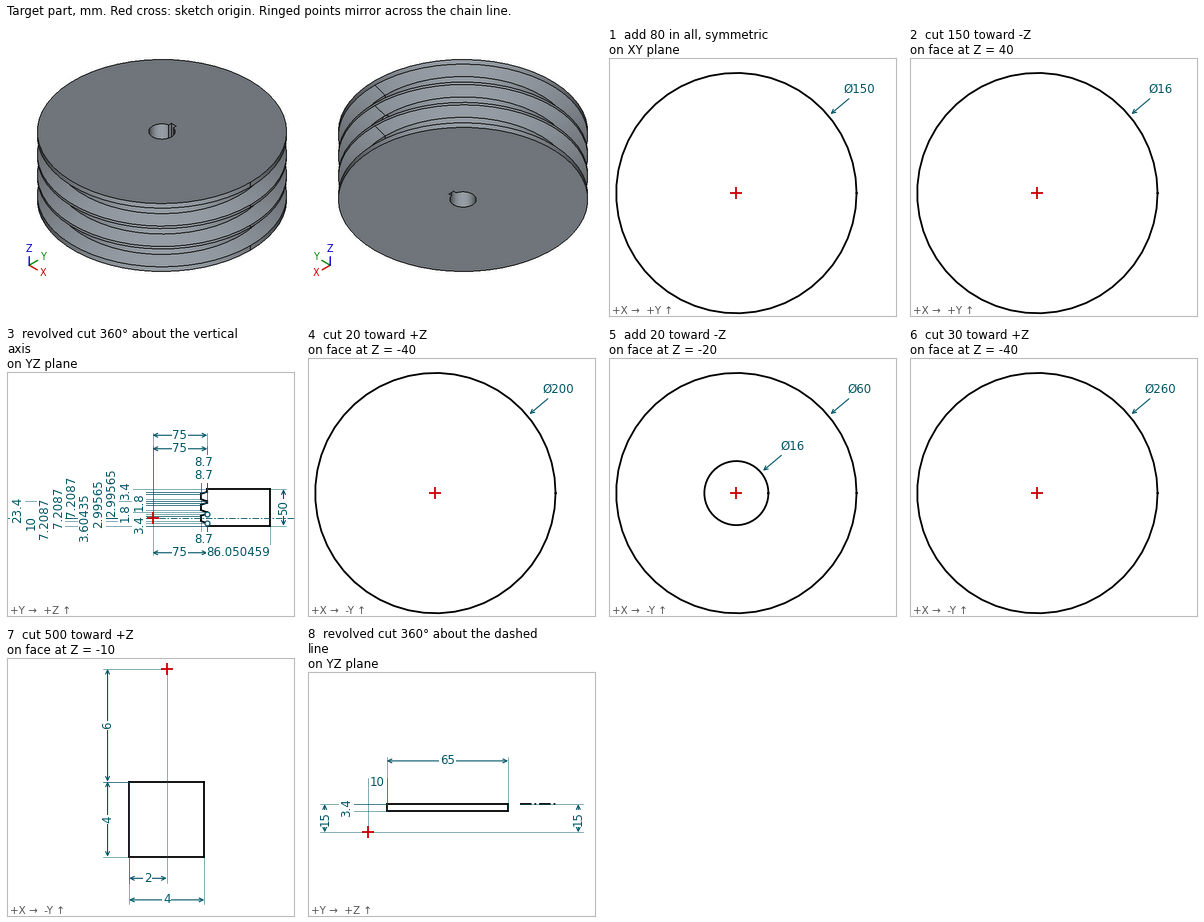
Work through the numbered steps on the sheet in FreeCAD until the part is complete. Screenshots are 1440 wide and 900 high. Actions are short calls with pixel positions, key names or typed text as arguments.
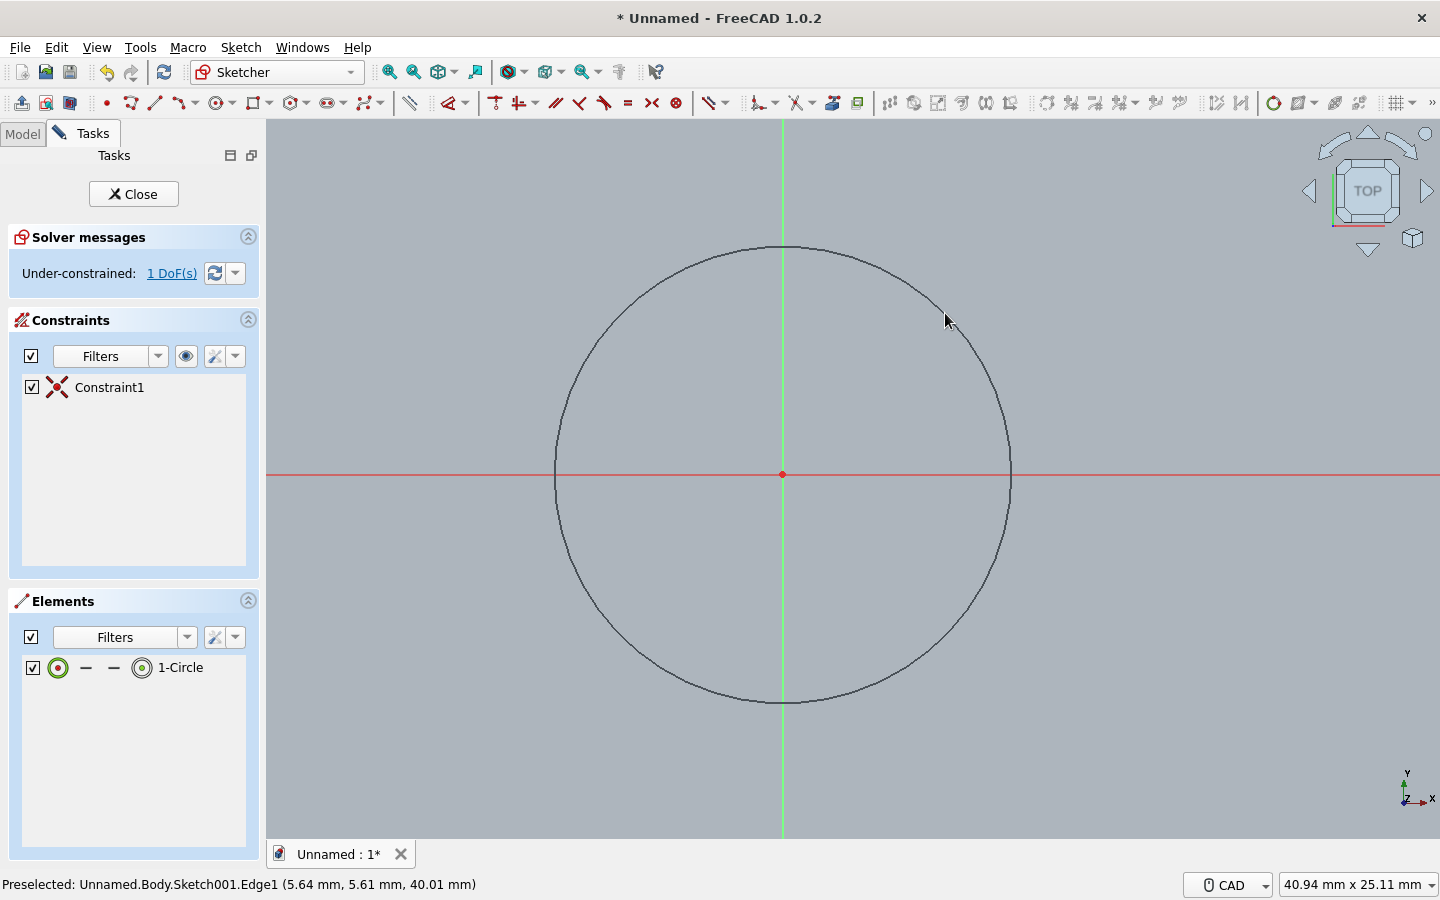
key(d)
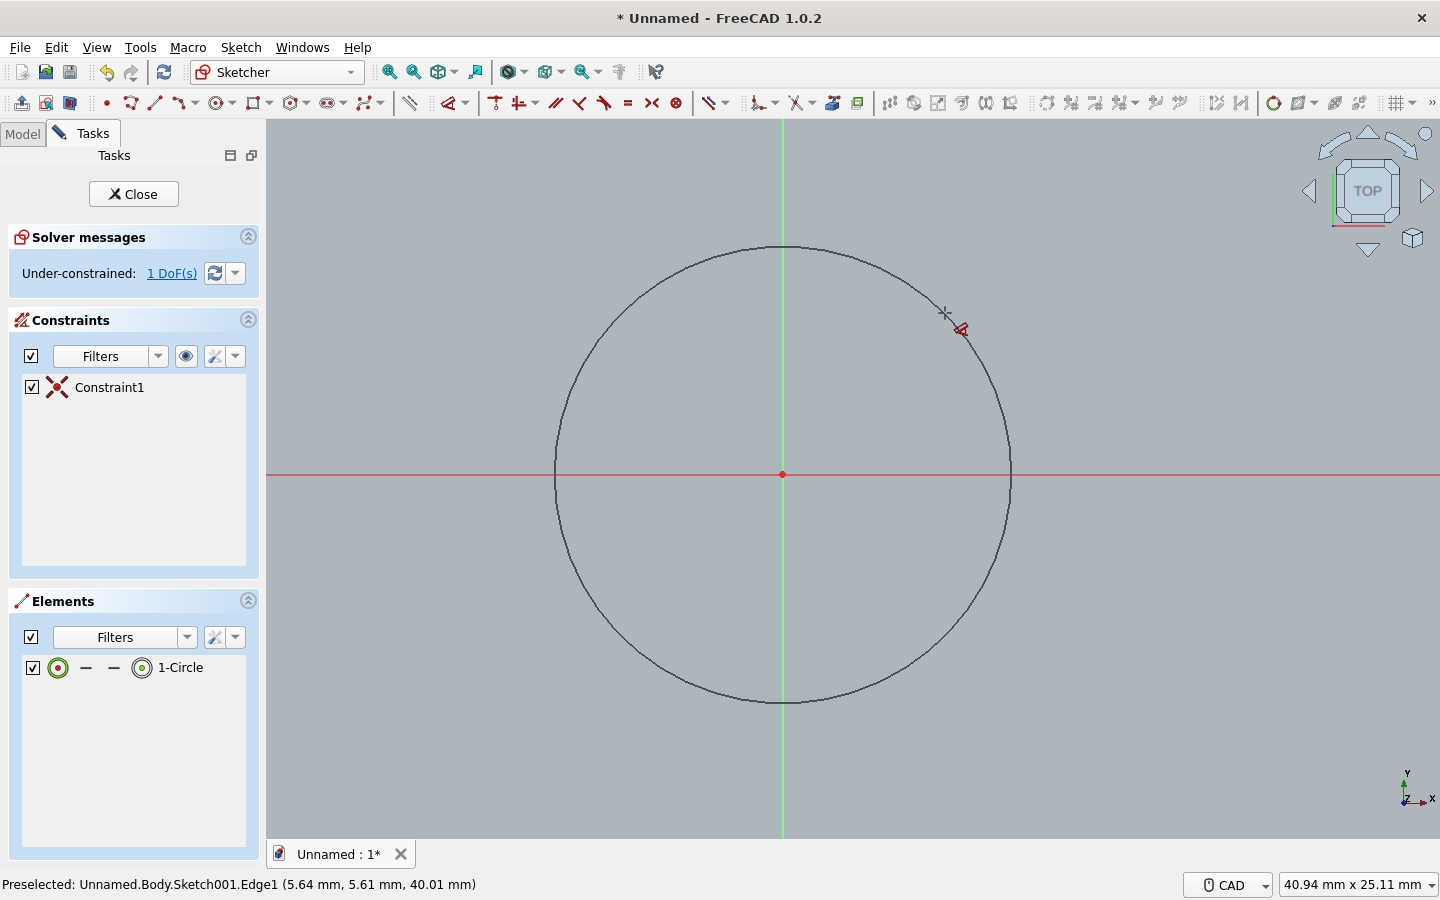
click(944, 313)
click(967, 290)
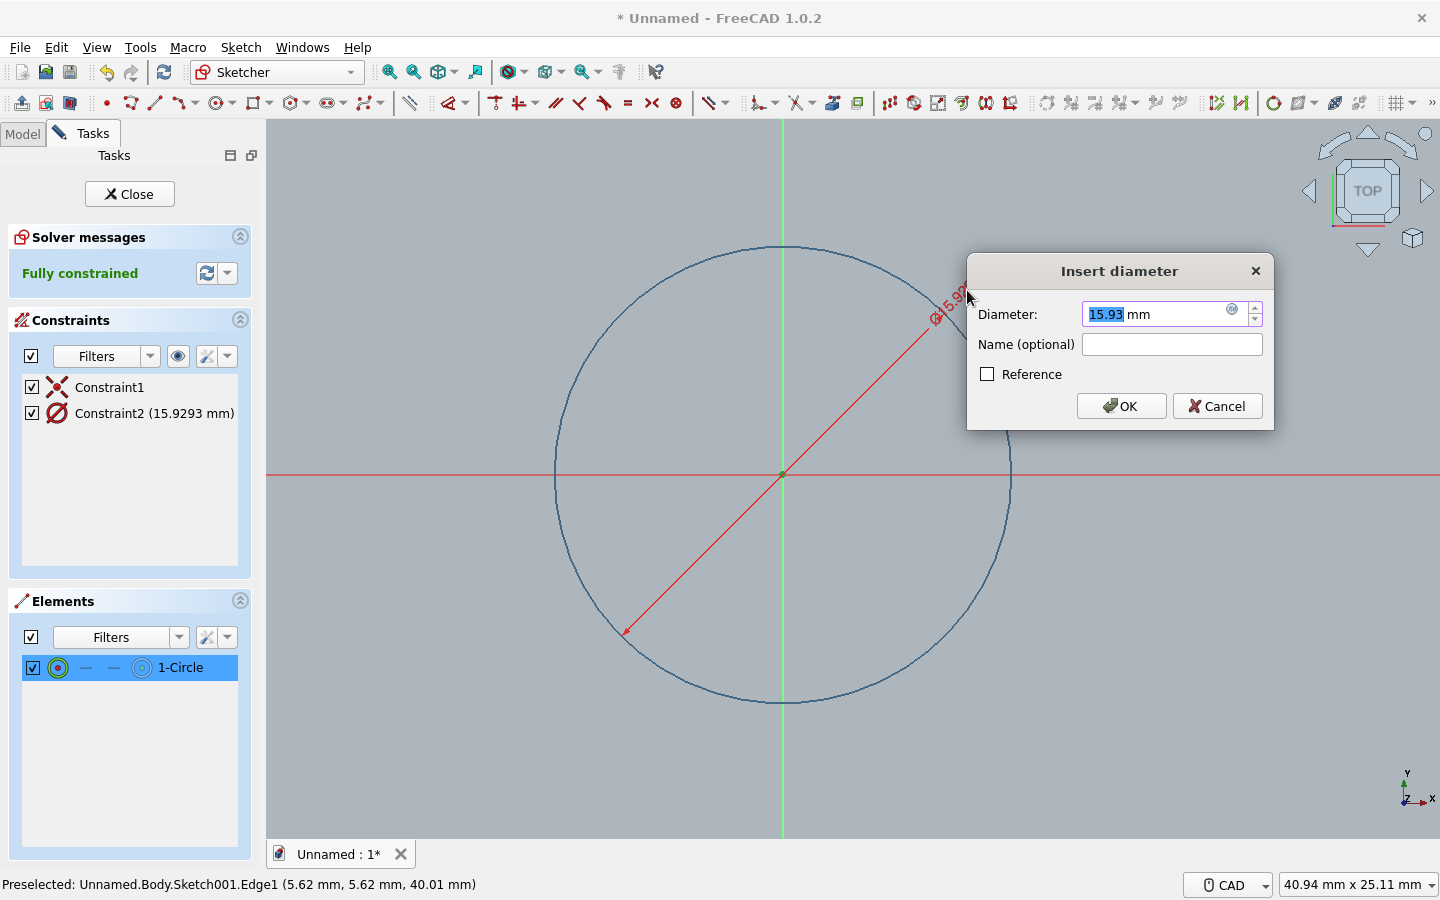
text(16)
key(Return)
key(Escape)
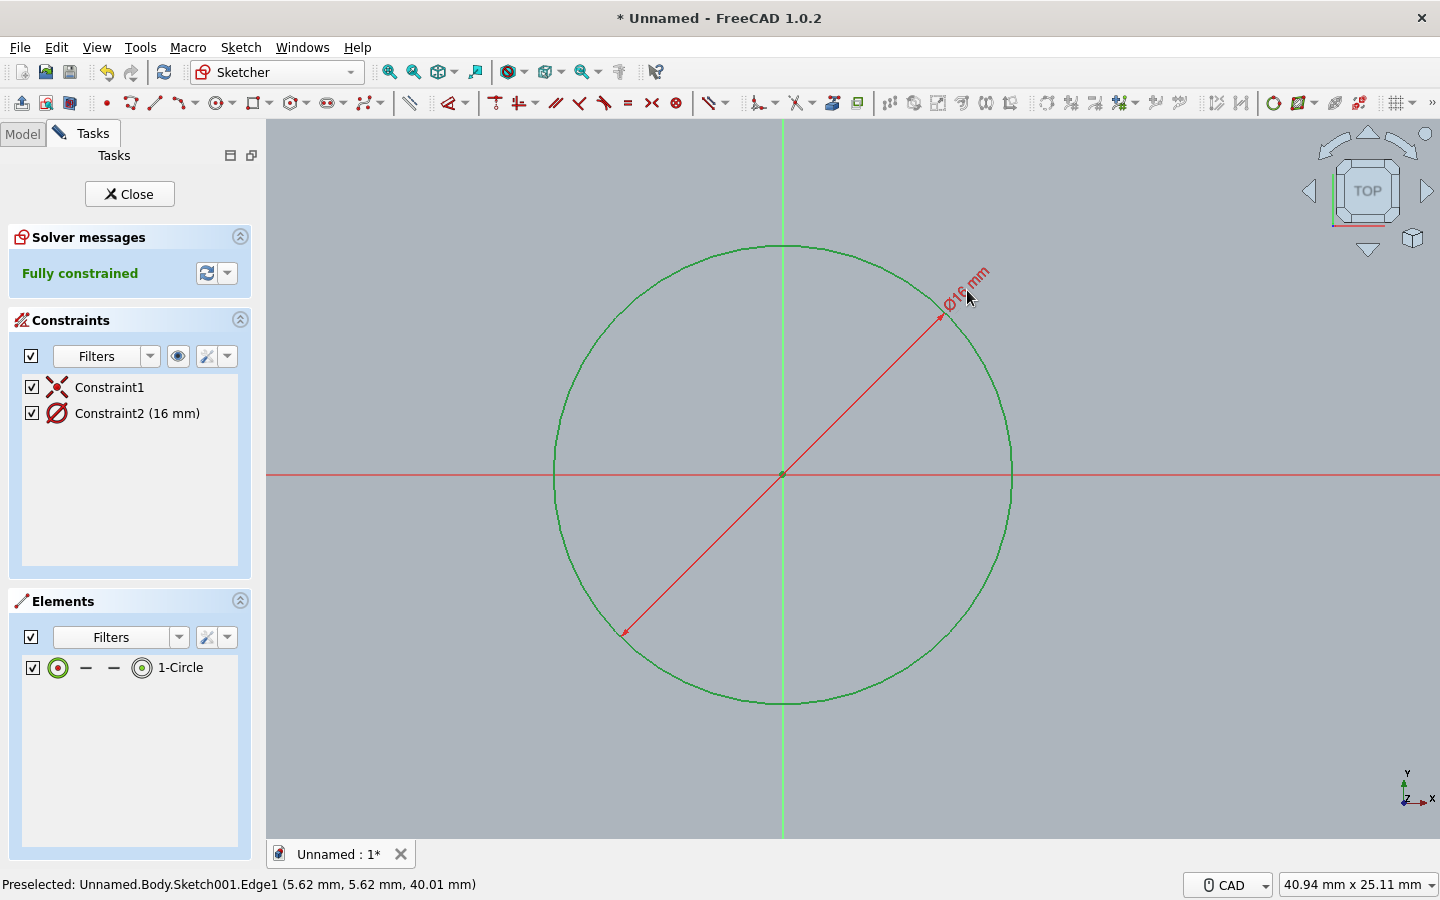
click(130, 194)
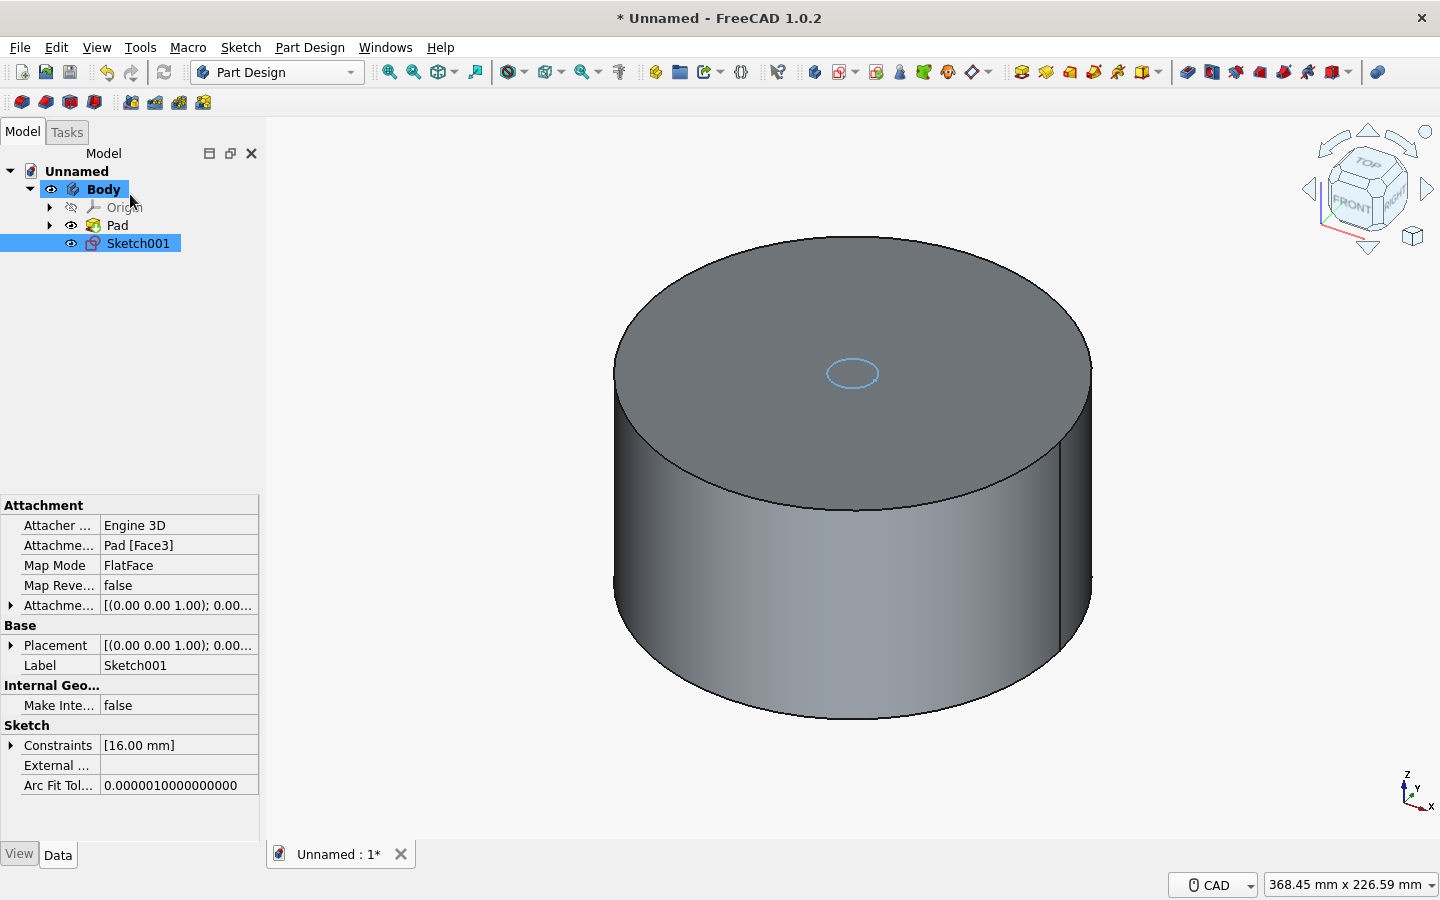
click(1188, 72)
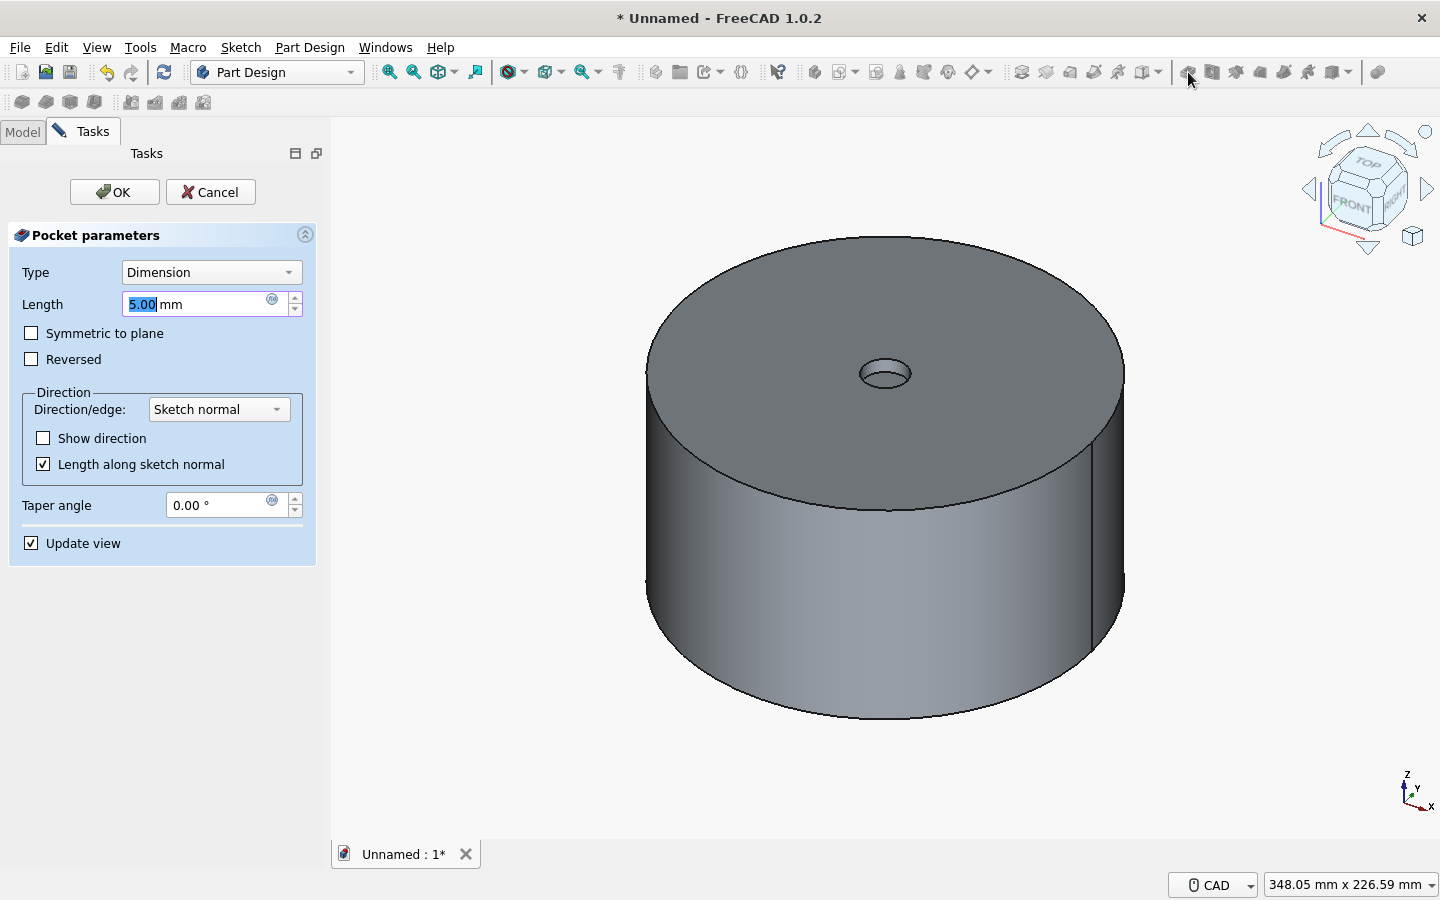
text(150)
key(Tab)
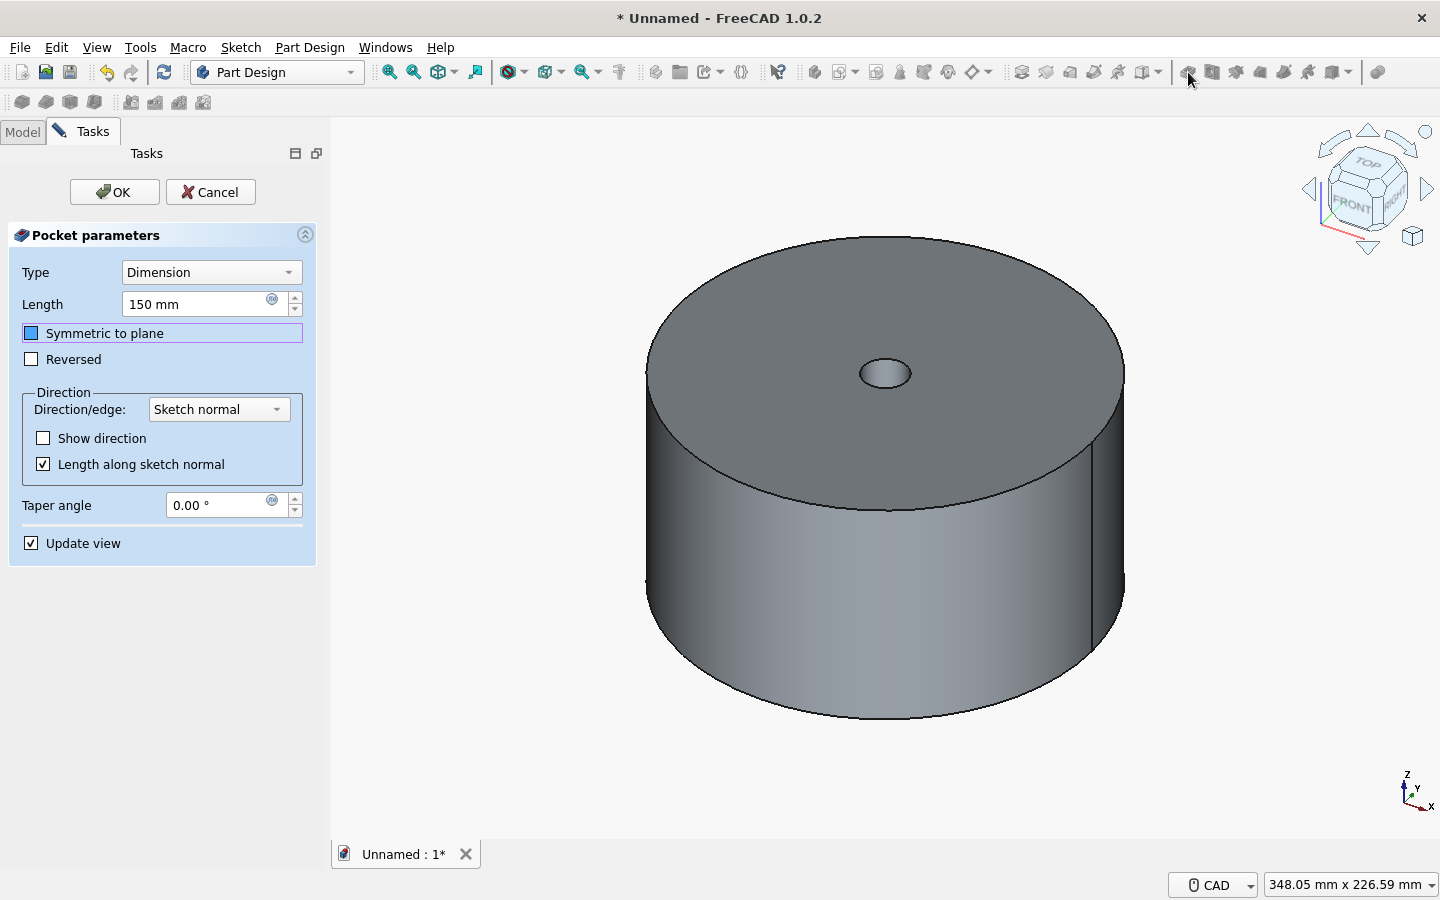
click(115, 192)